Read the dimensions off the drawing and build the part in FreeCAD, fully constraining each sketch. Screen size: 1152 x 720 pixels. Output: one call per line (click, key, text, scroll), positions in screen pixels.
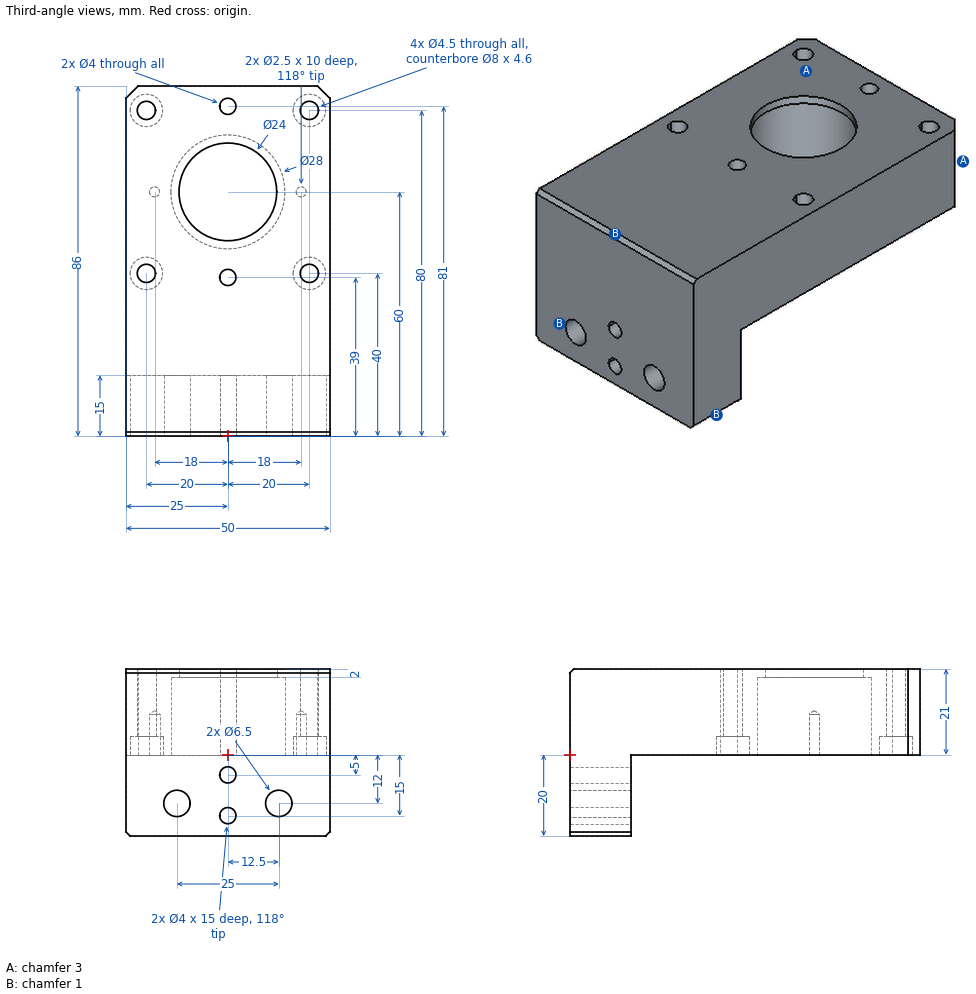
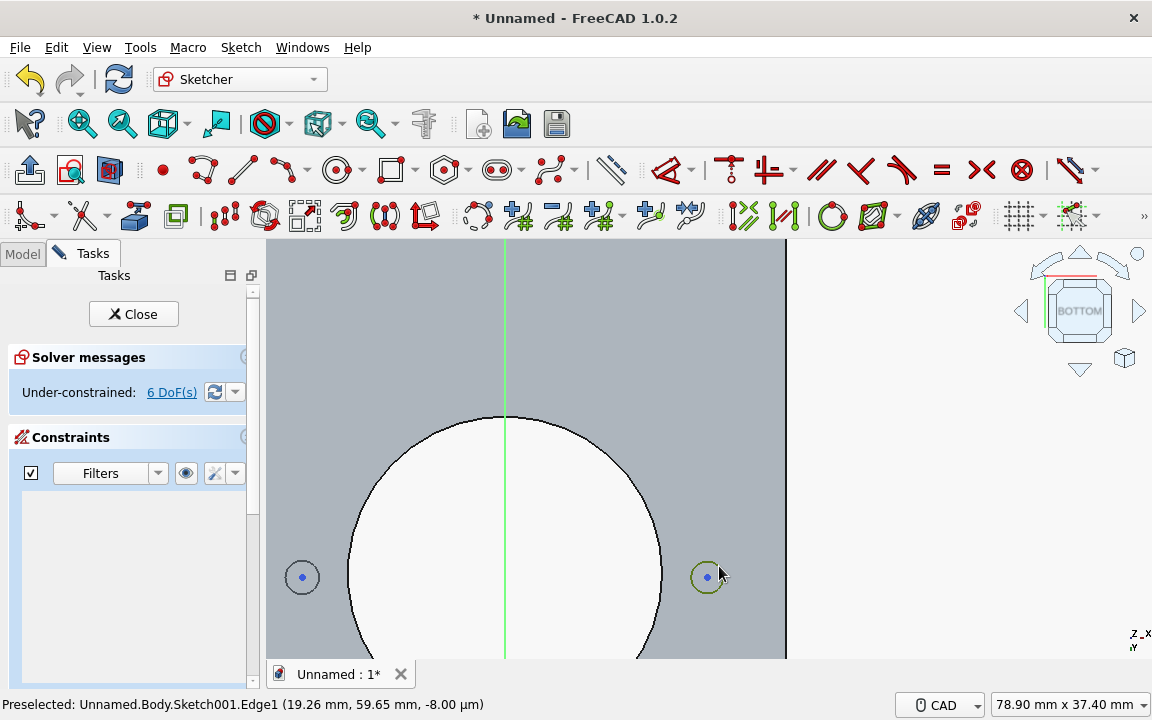
click(314, 566)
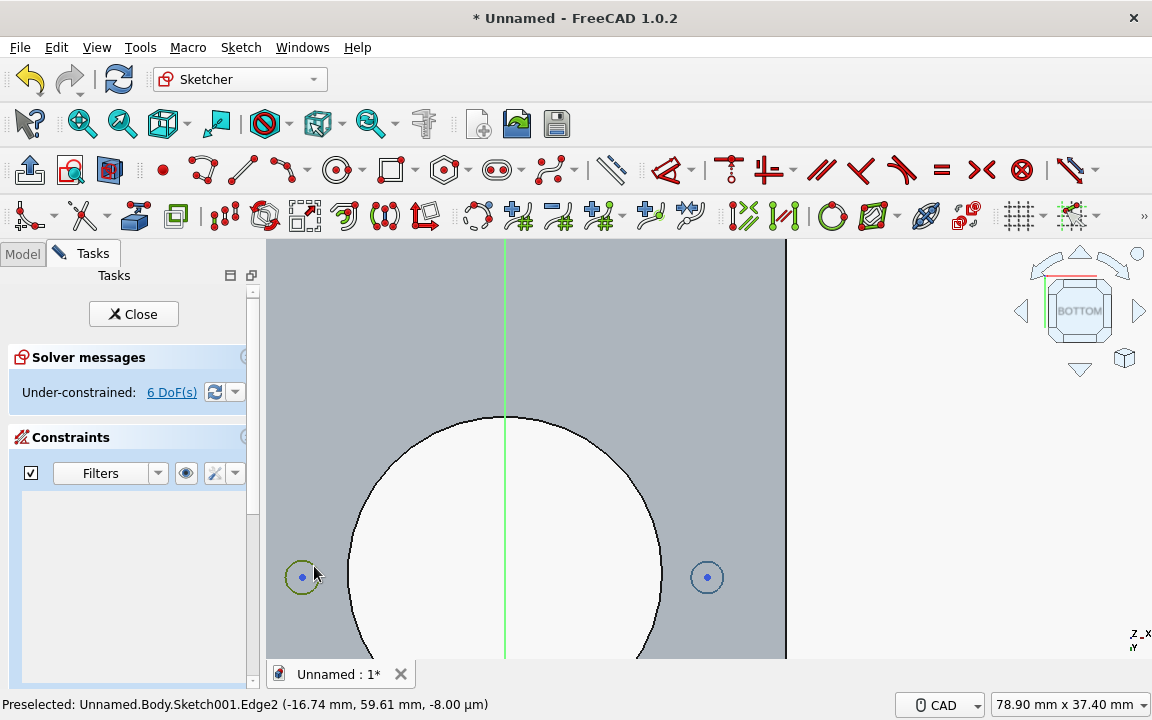
click(942, 170)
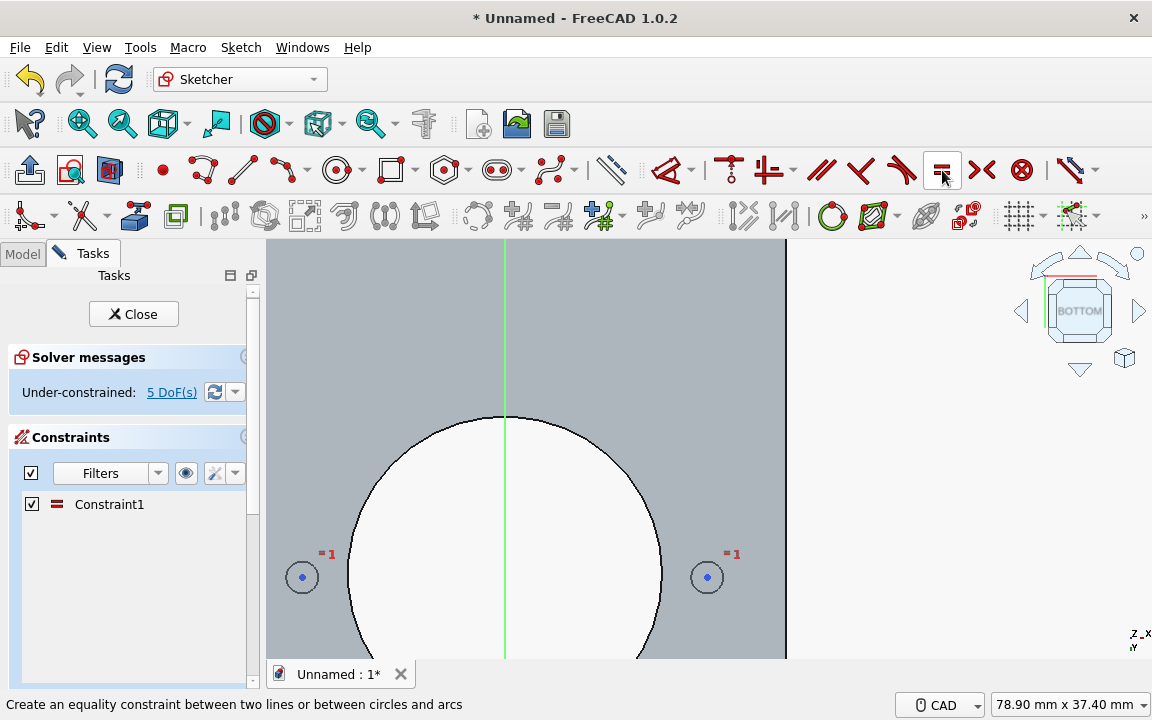
click(707, 578)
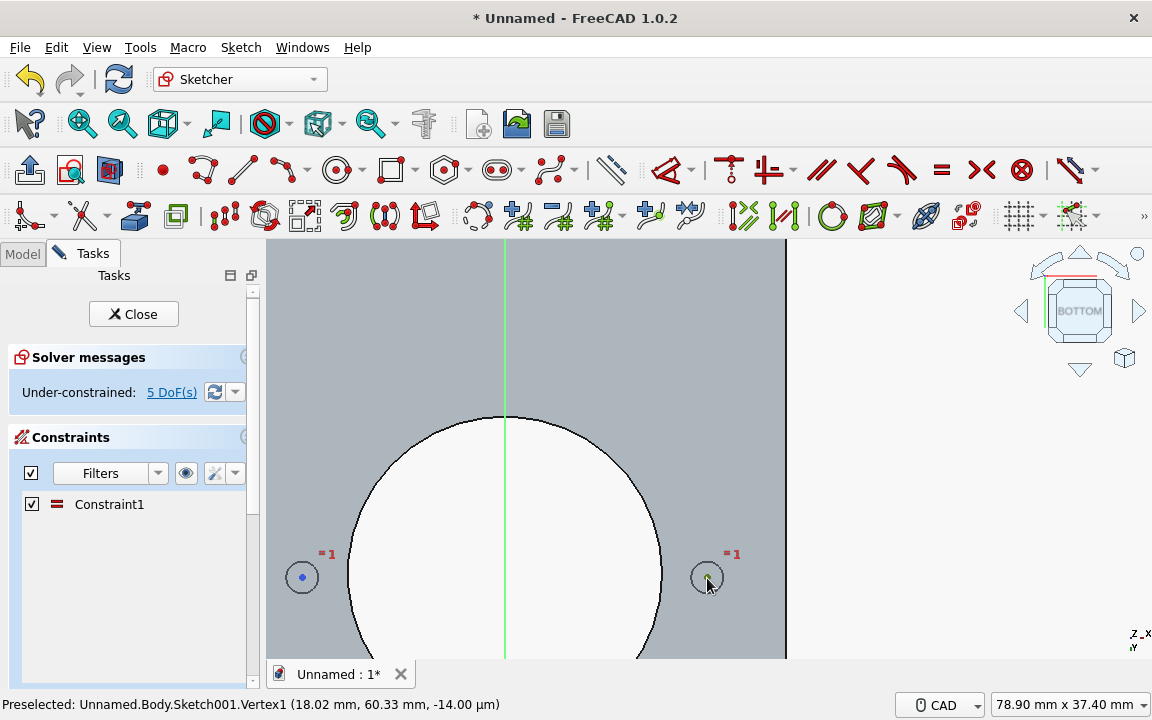
click(302, 578)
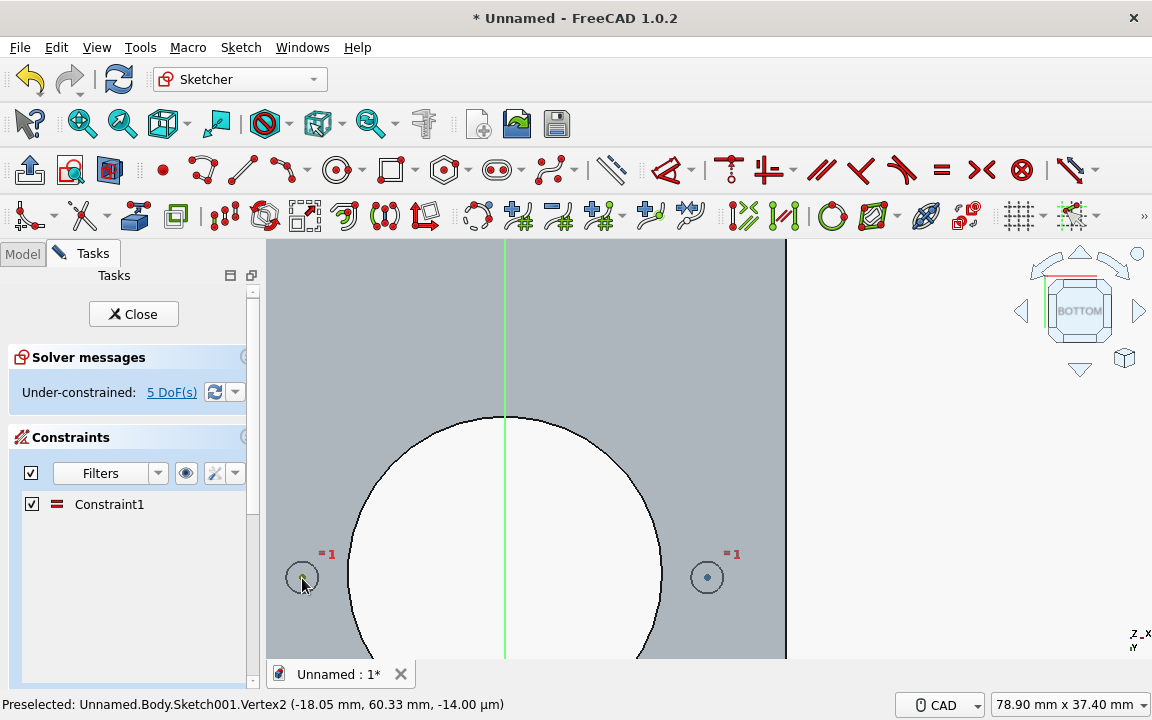
click(796, 170)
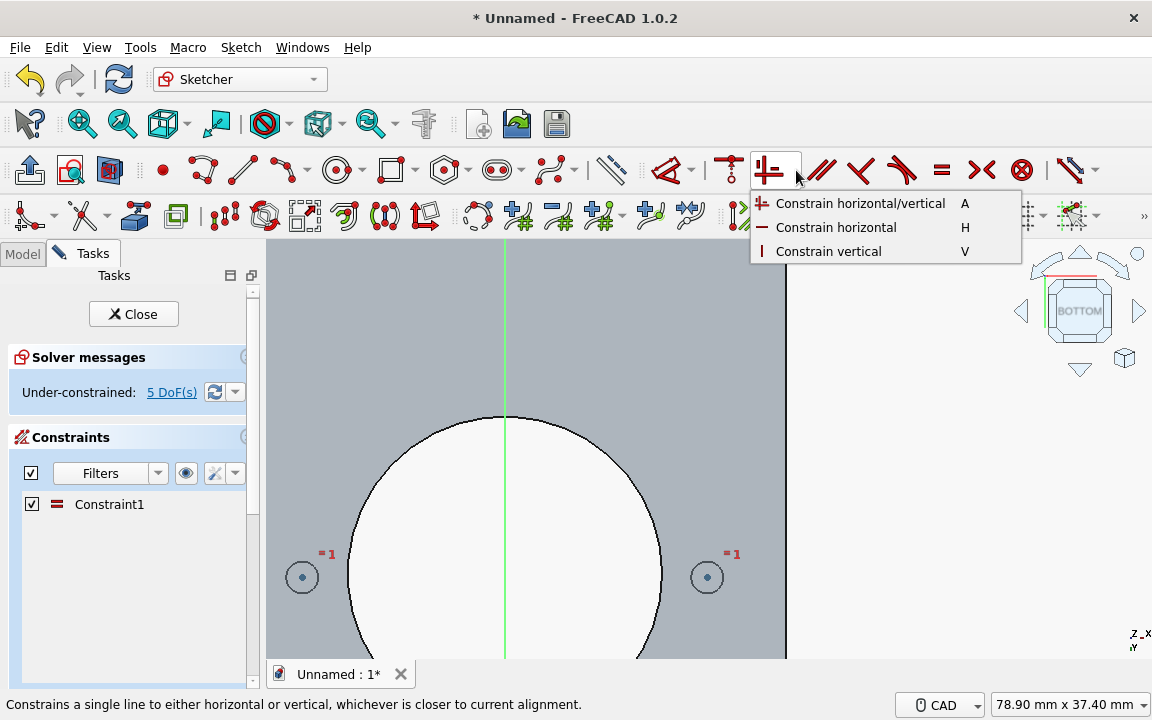
click(886, 227)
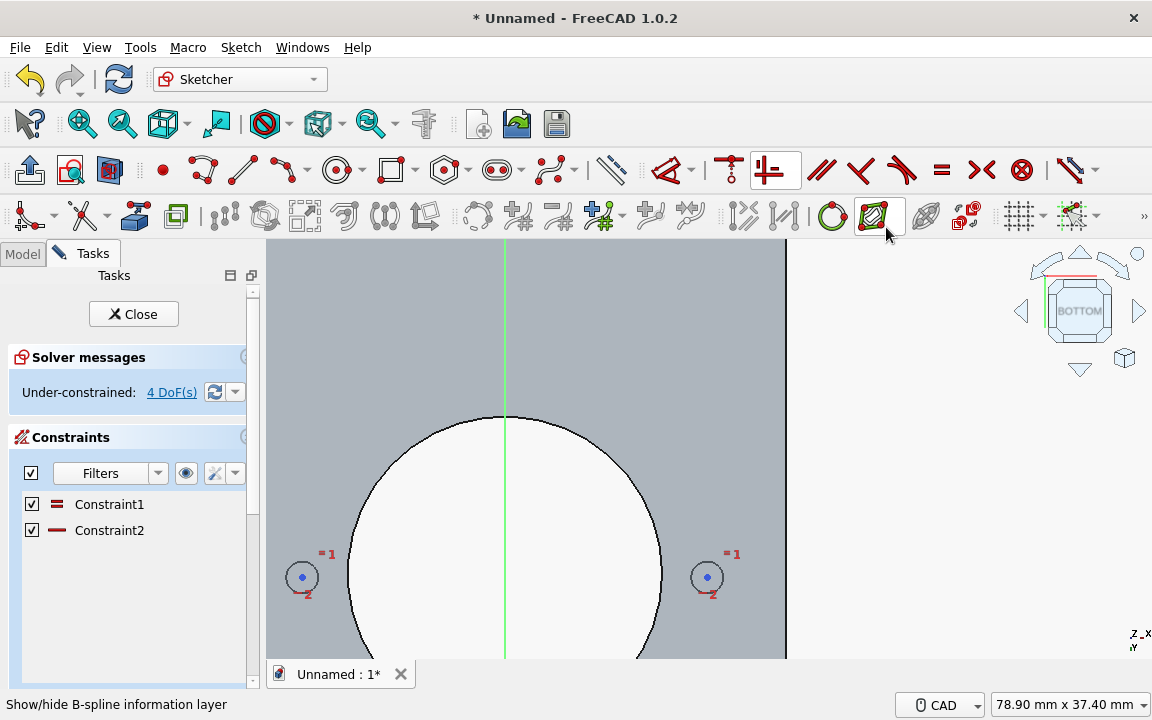
scroll(719, 566, up, 2)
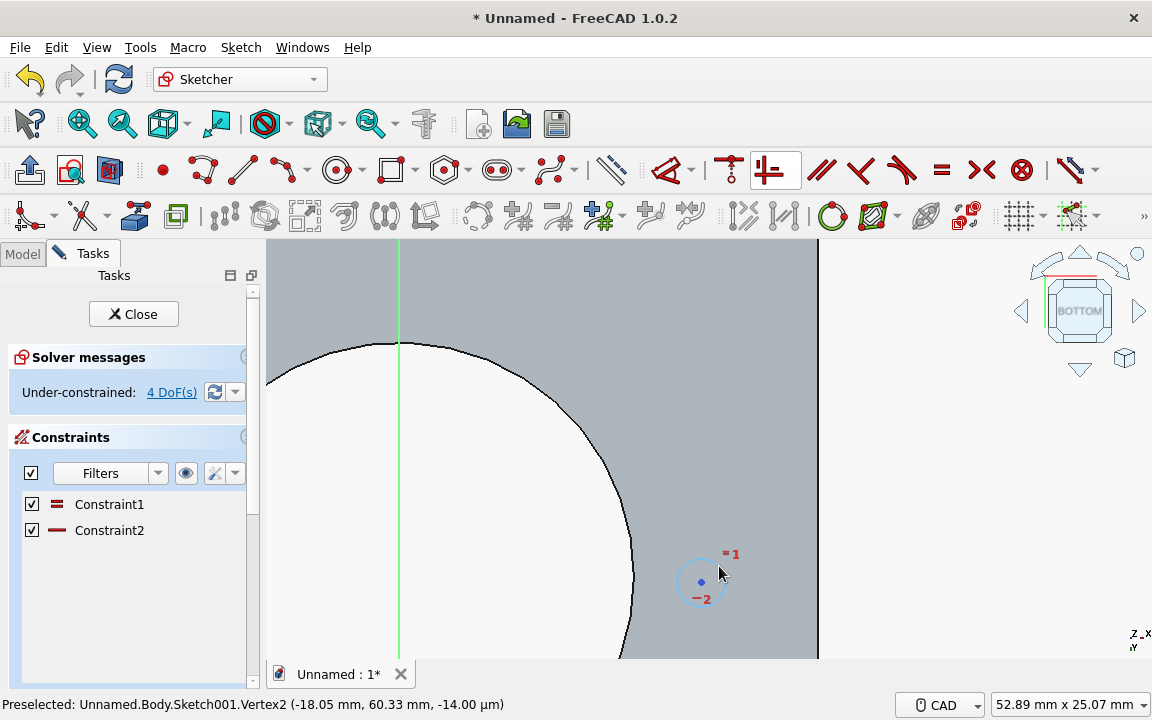
click(718, 566)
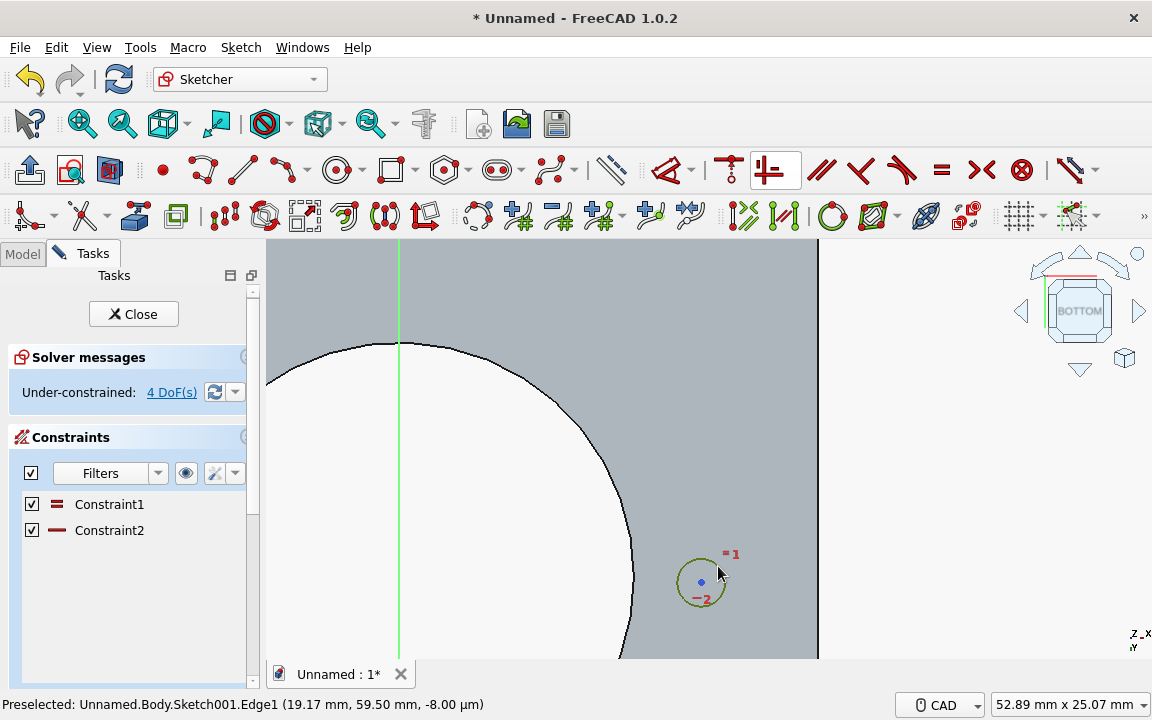
key(k)
key(o)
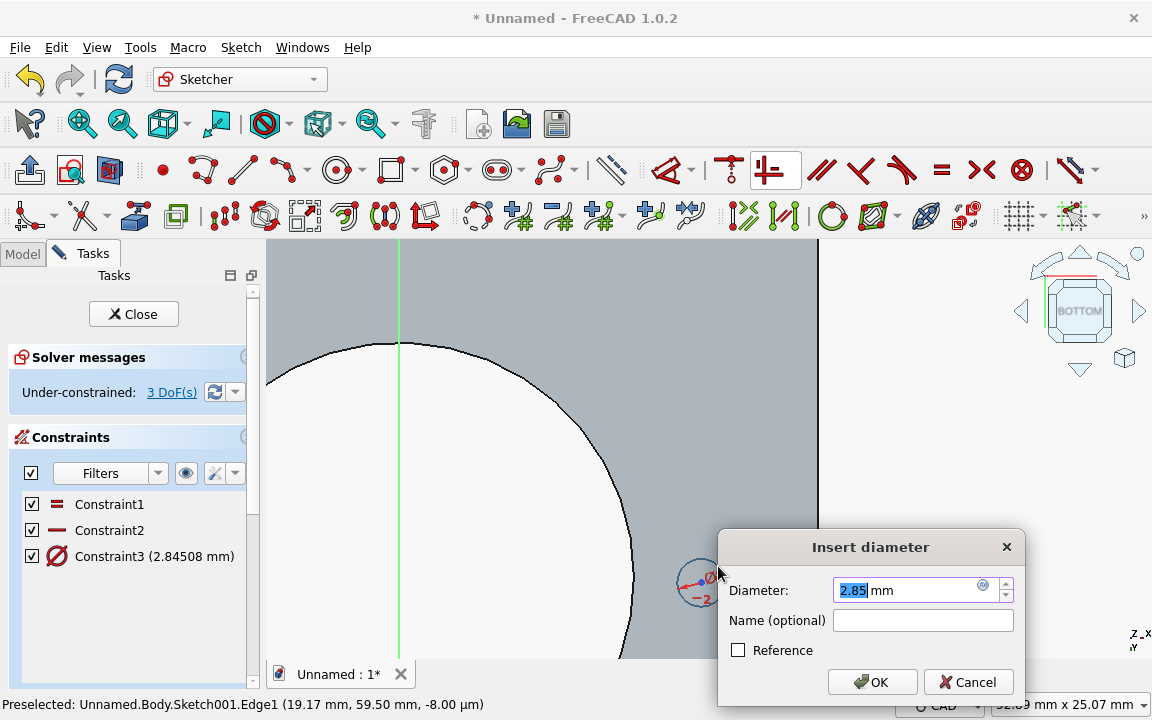
text(2.5)
key(Return)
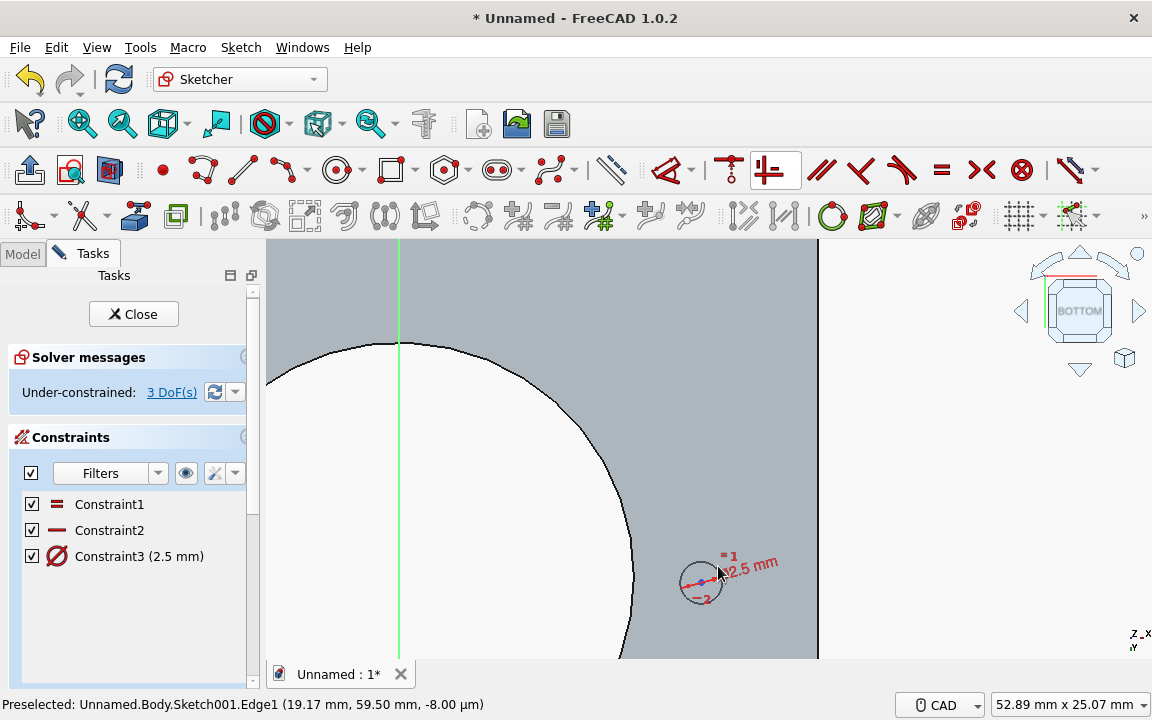
scroll(719, 568, down, 7)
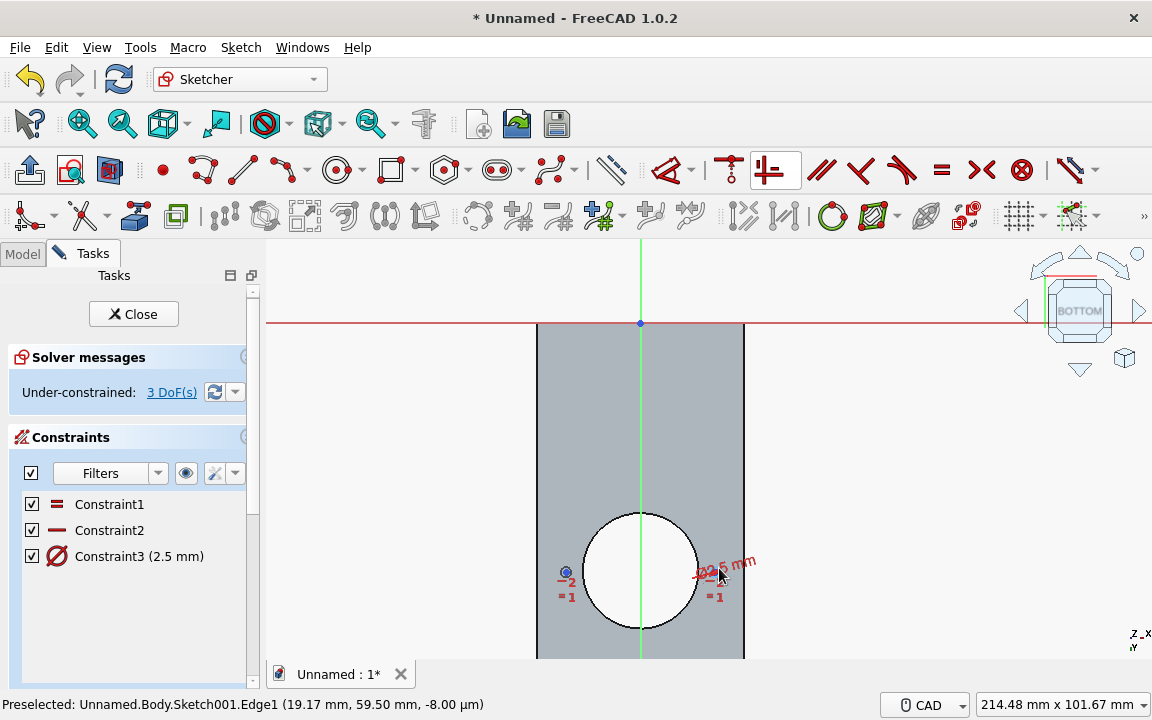
click(715, 572)